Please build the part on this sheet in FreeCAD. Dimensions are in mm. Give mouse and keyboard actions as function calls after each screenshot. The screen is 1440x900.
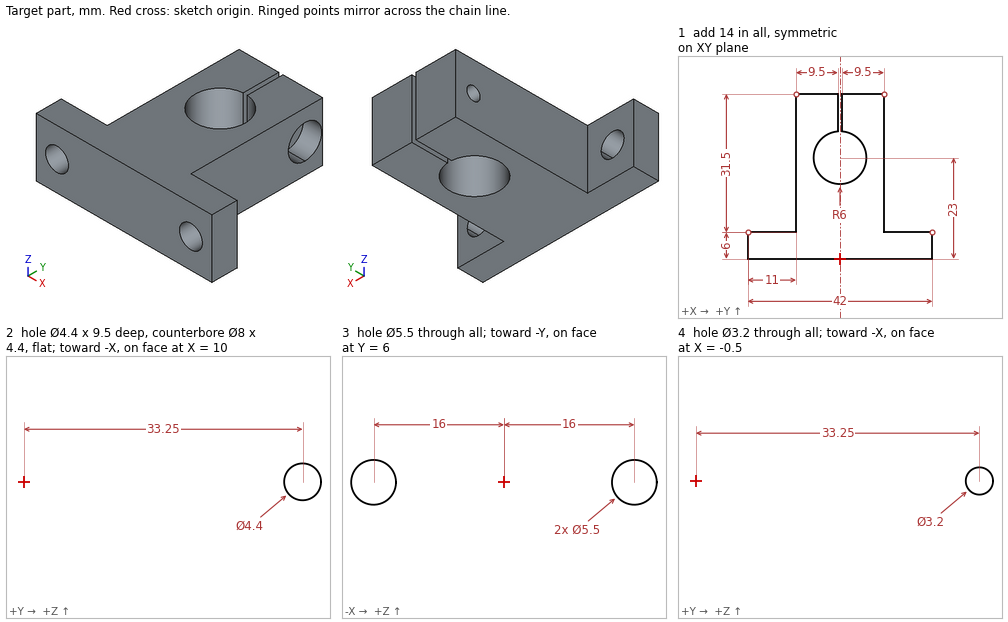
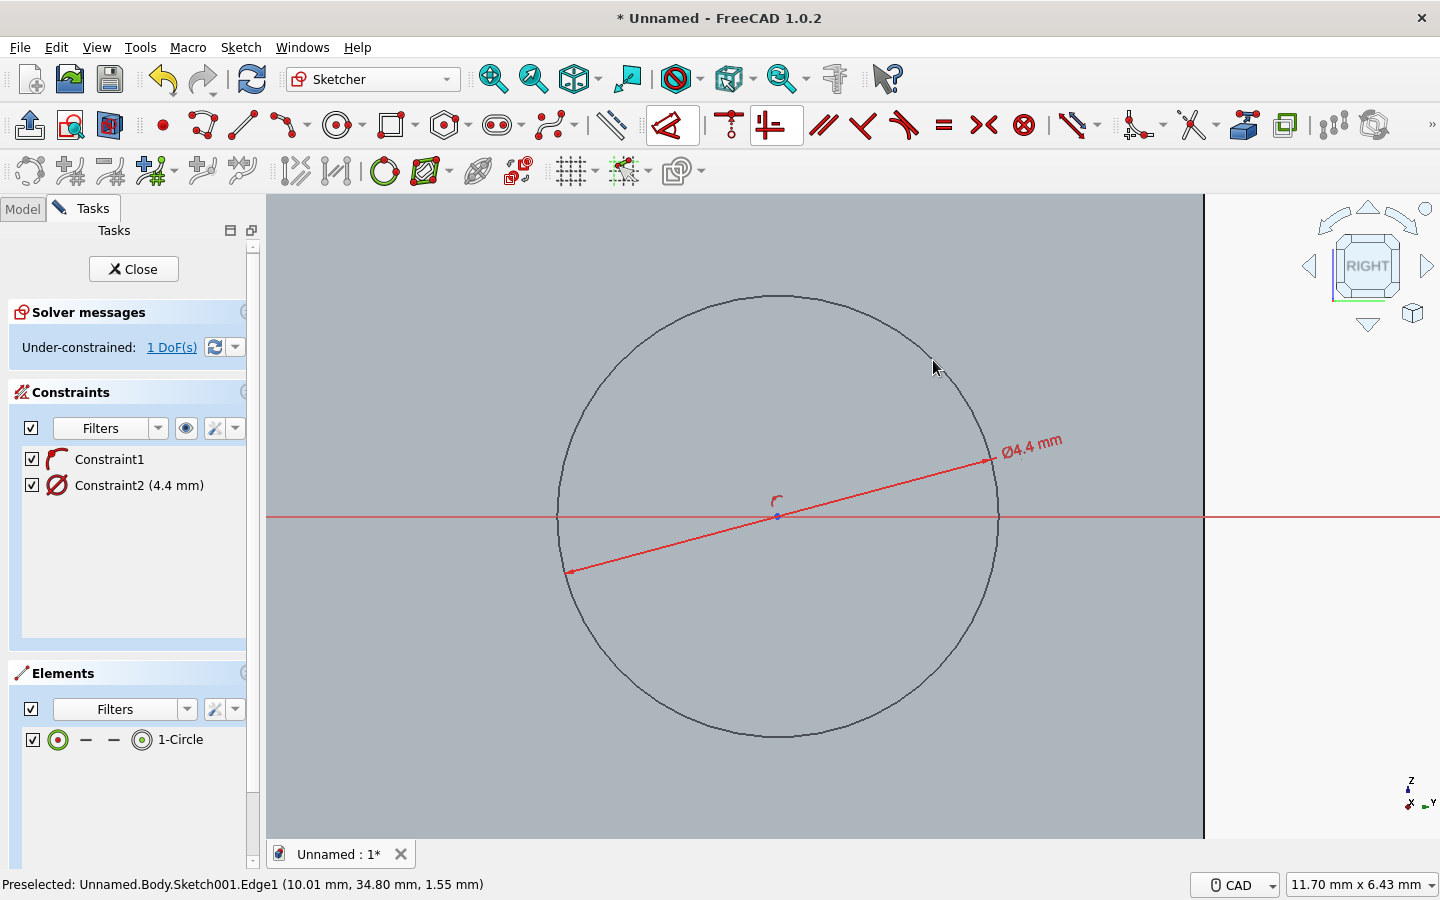
click(778, 516)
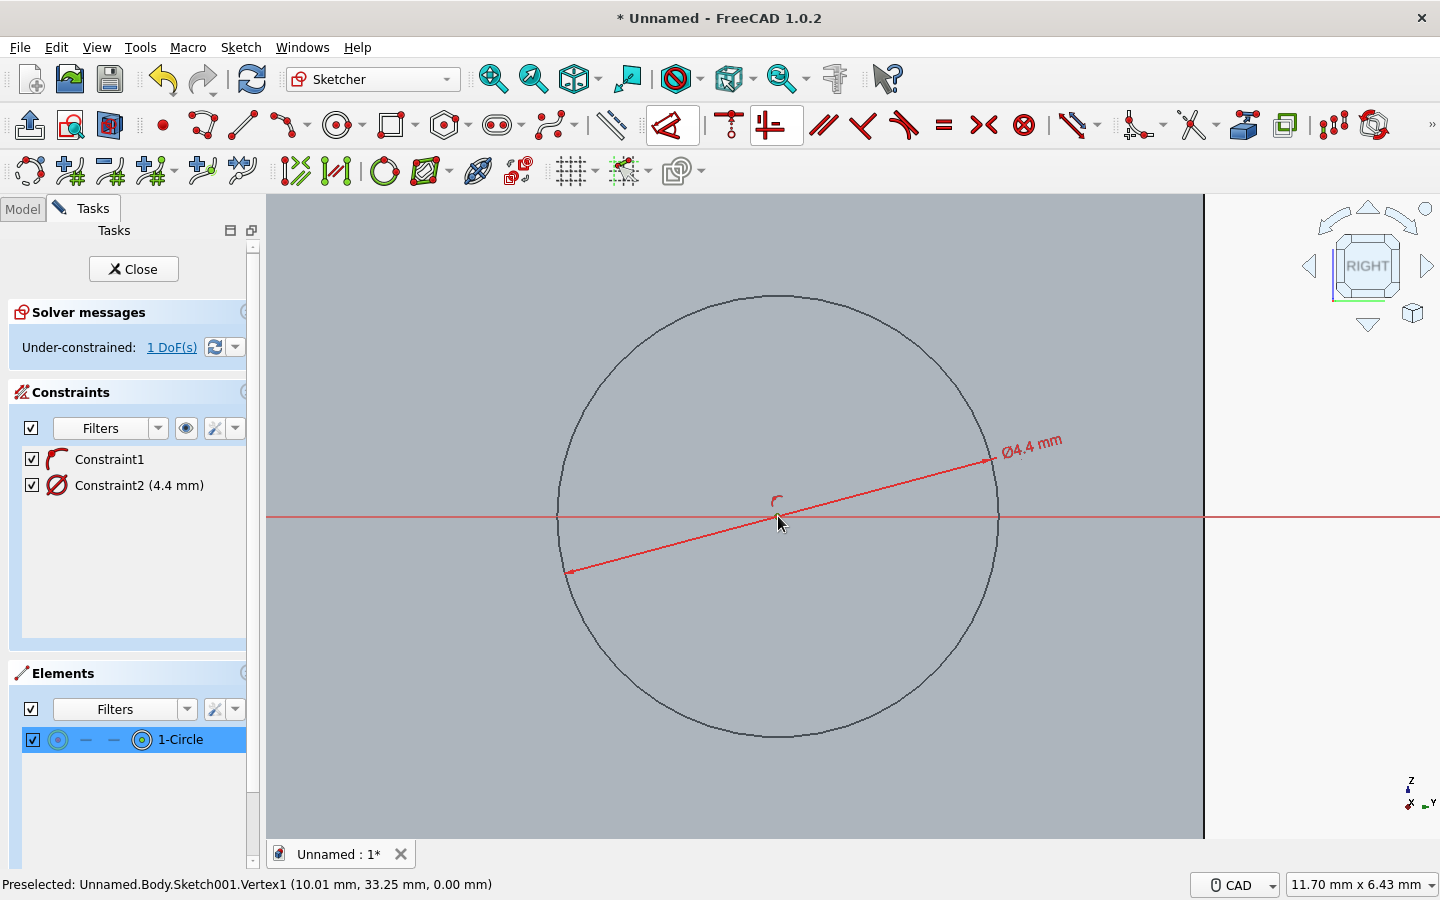
click(694, 126)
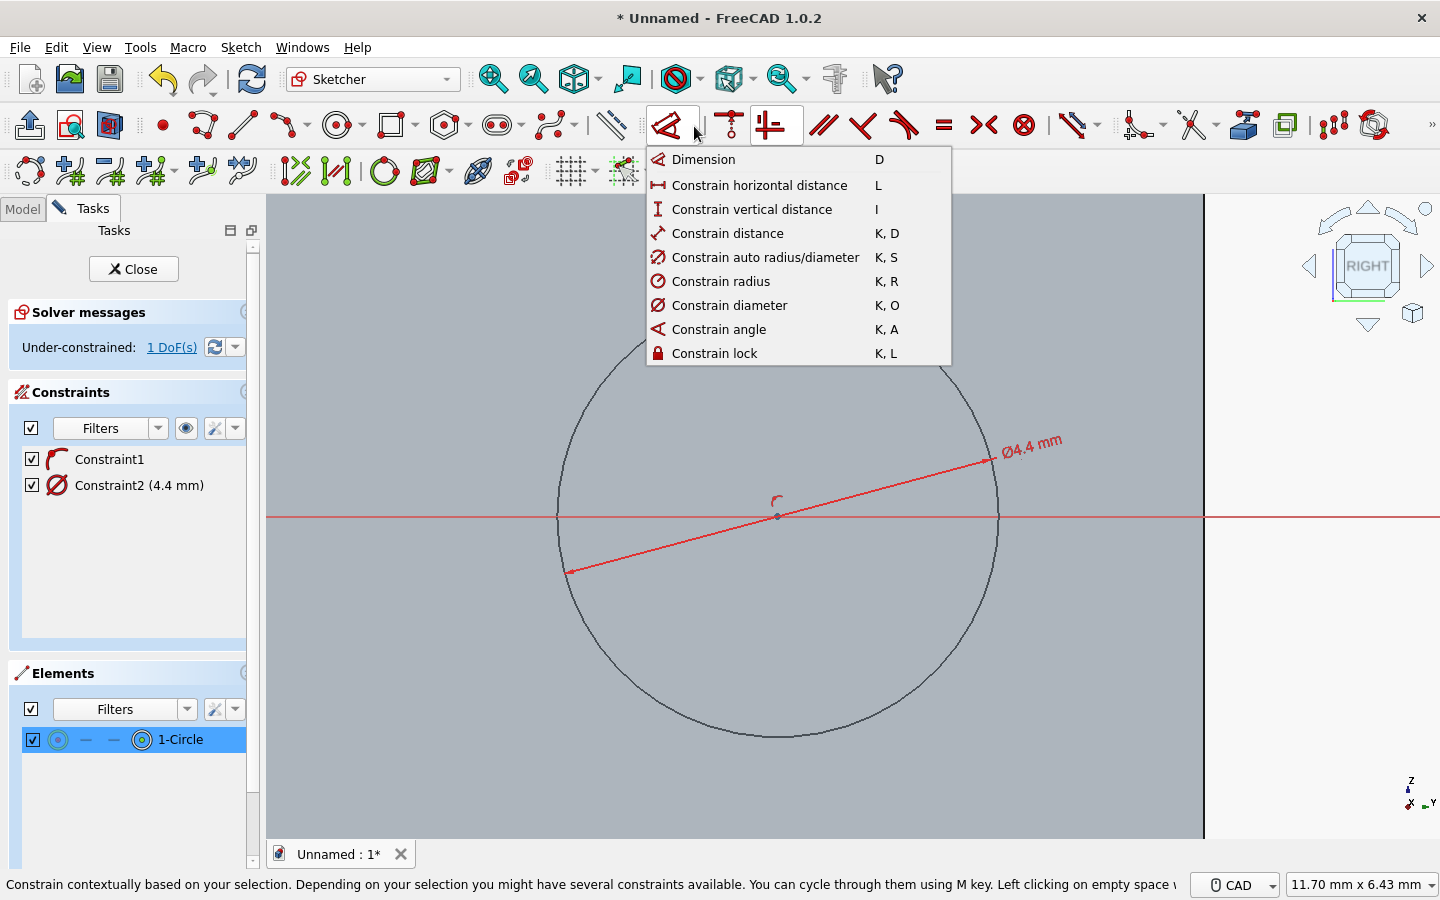
click(799, 185)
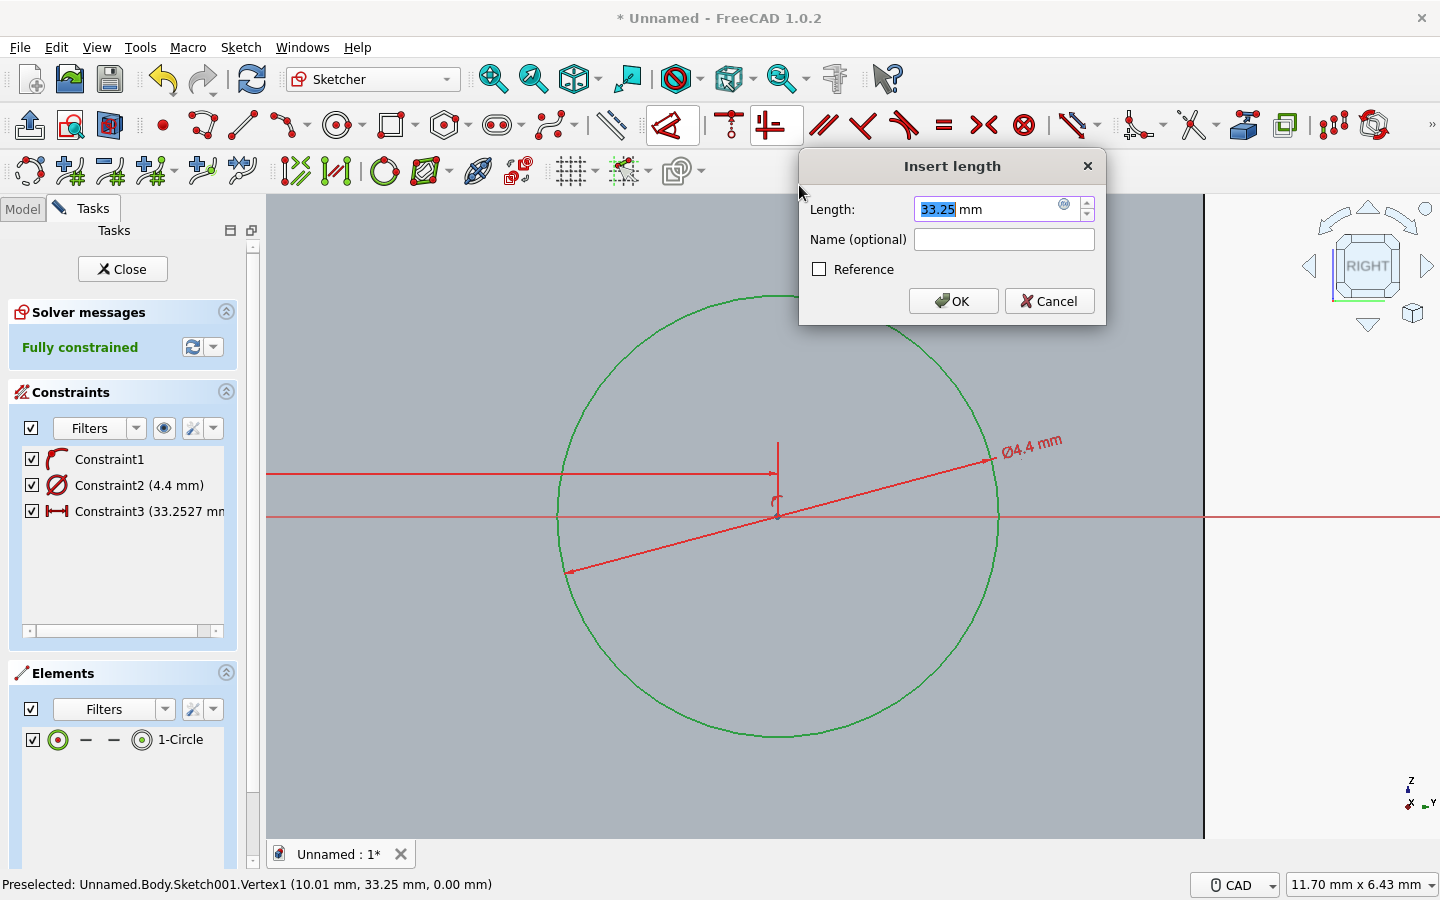
text(33.25)
key(Return)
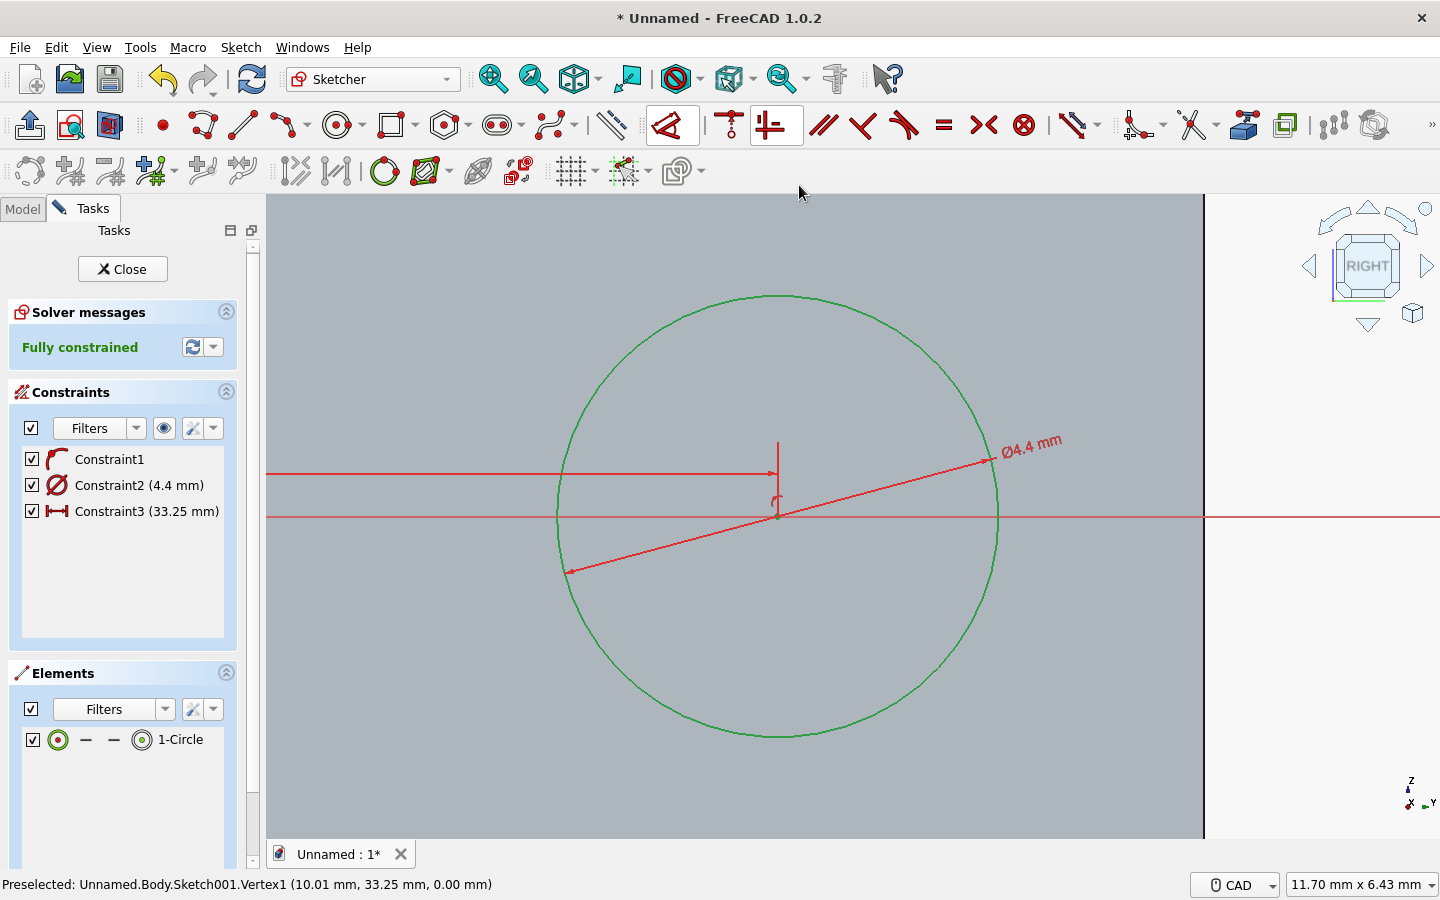
click(123, 269)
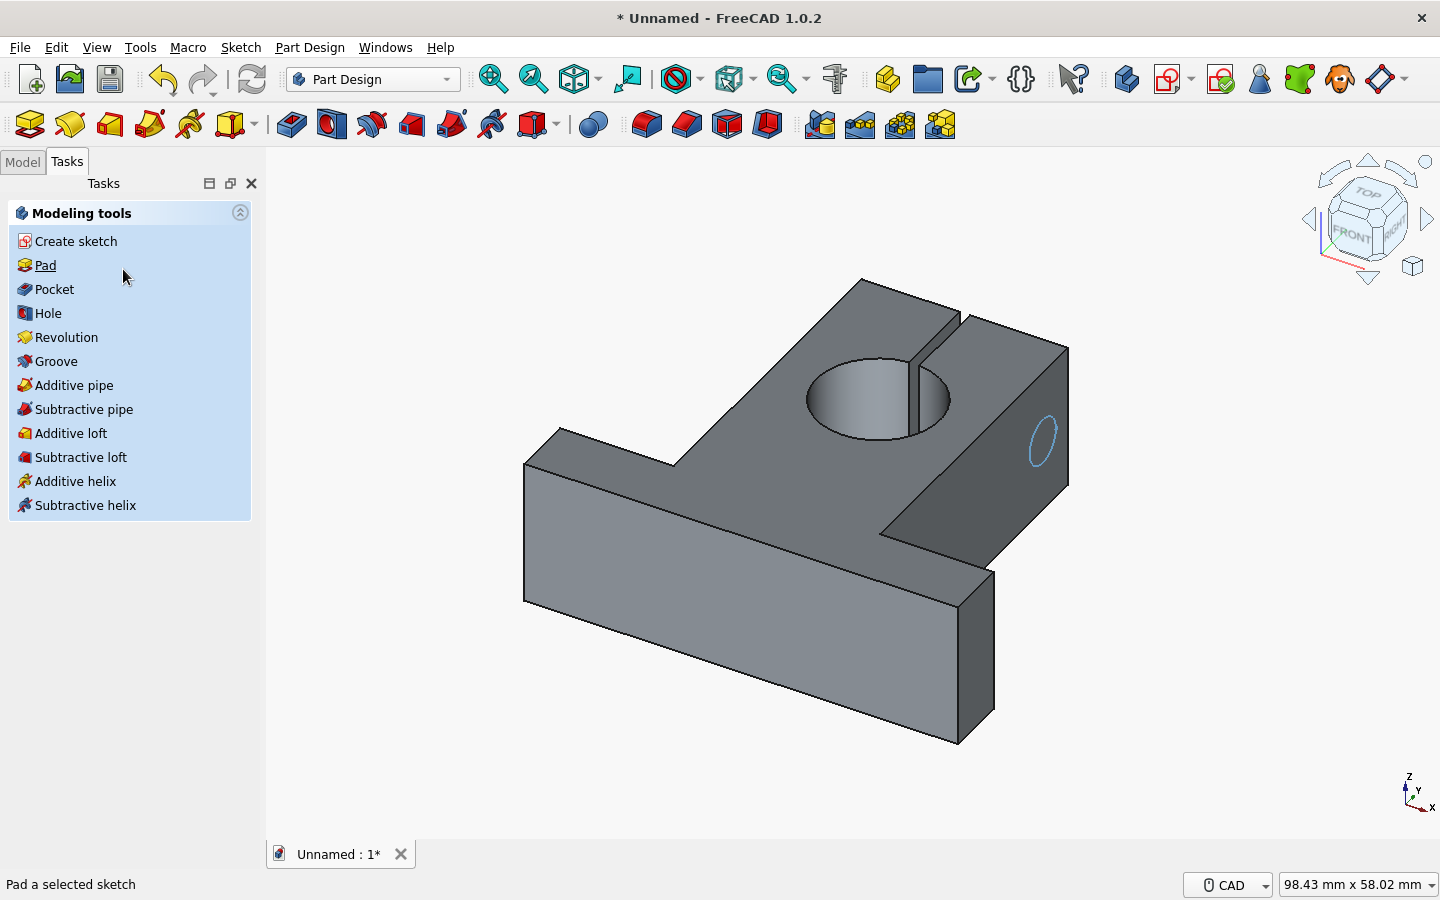
click(332, 124)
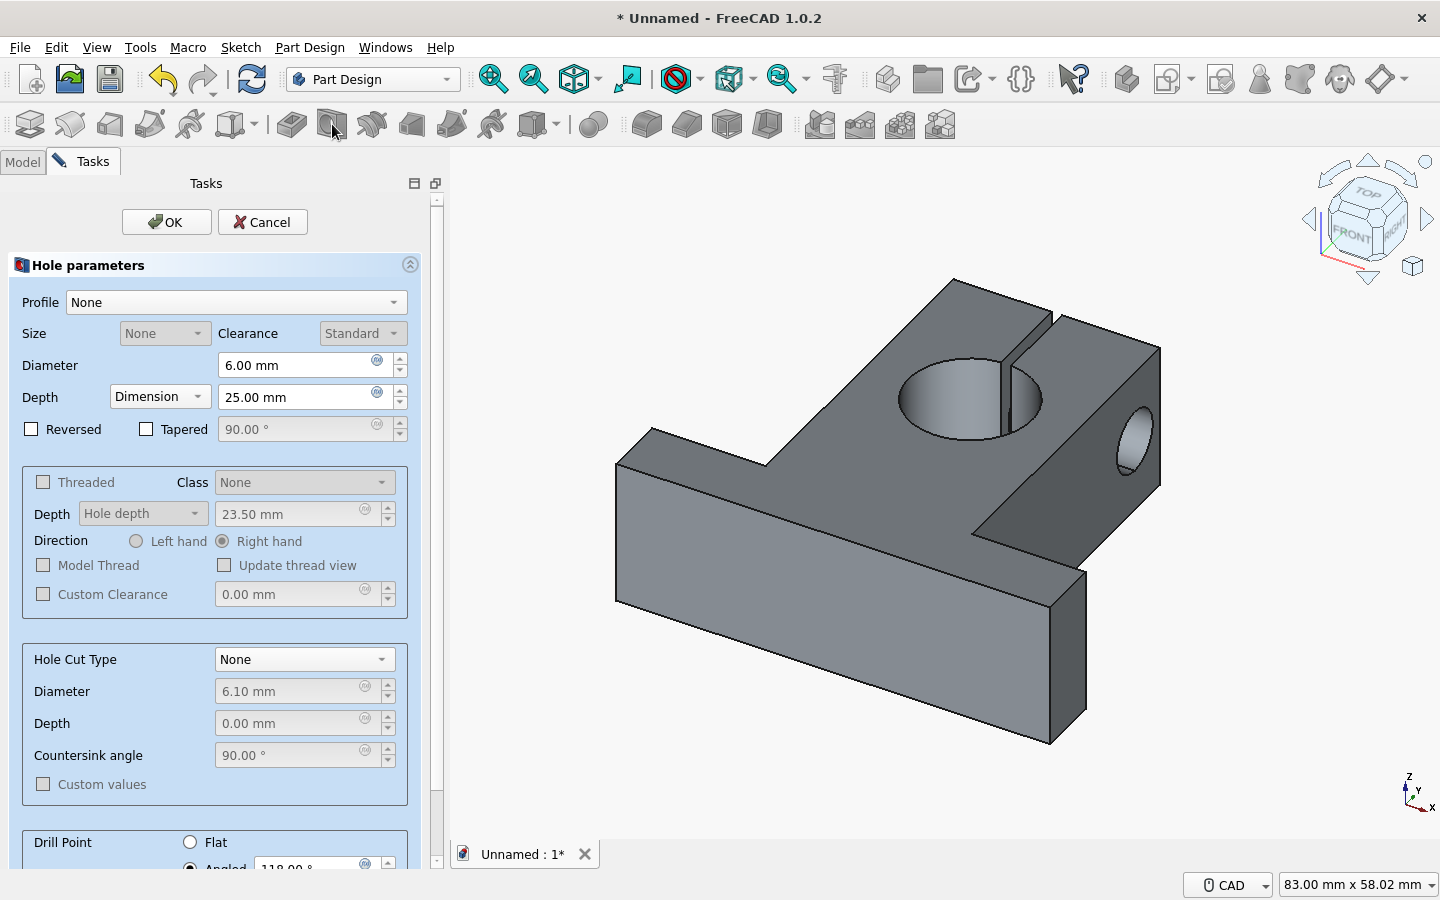
triple_click(305, 365)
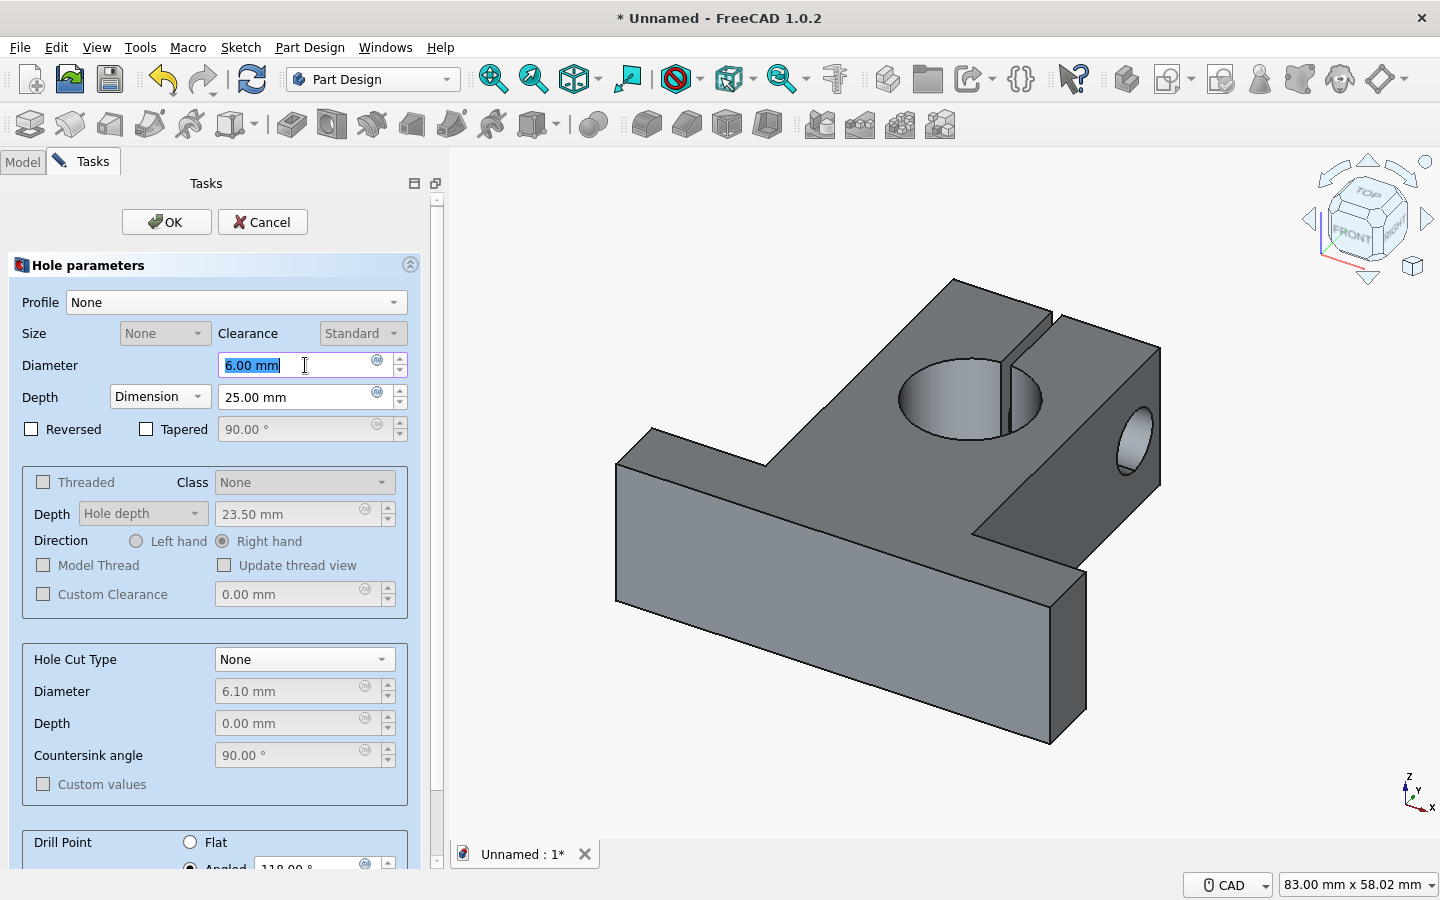
text(4.4)
key(Tab)